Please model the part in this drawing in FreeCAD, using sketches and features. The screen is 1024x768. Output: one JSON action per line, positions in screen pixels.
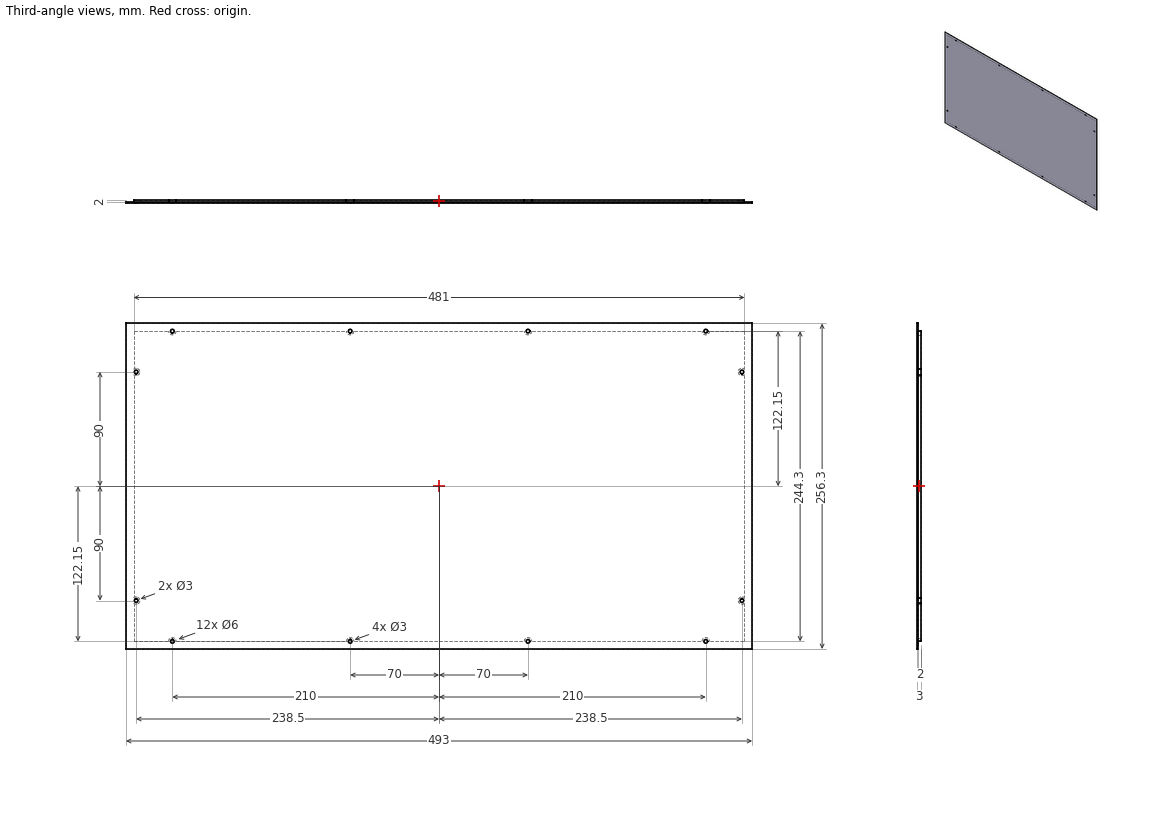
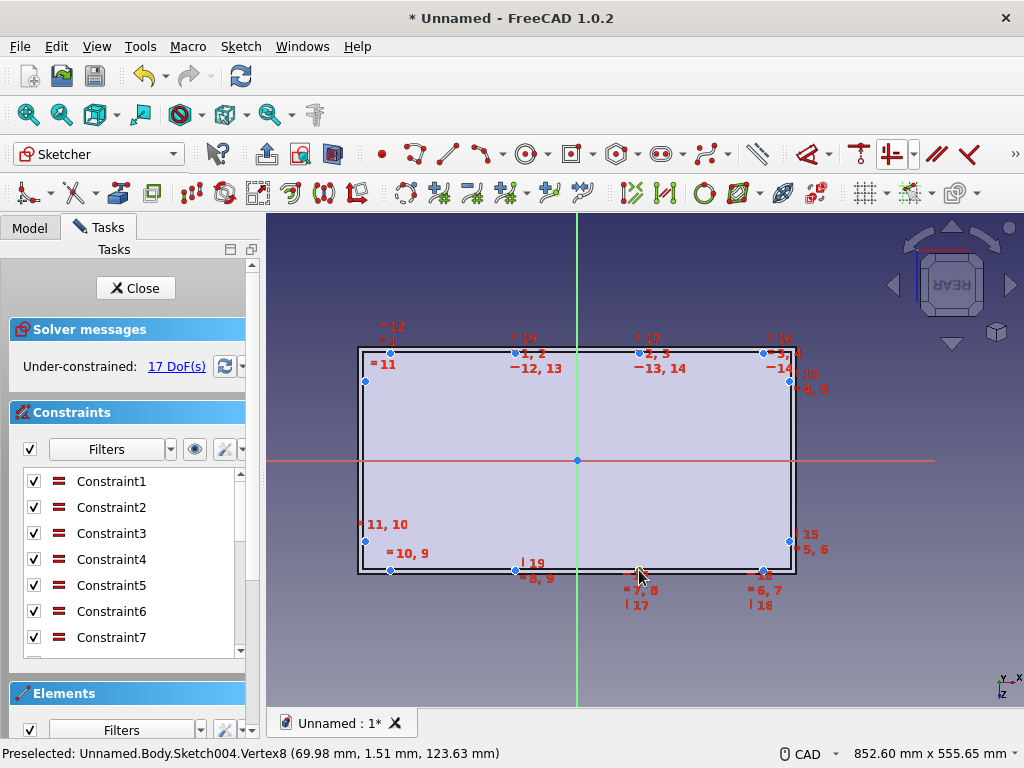
{"action": "left_click", "coordinate": [515, 570]}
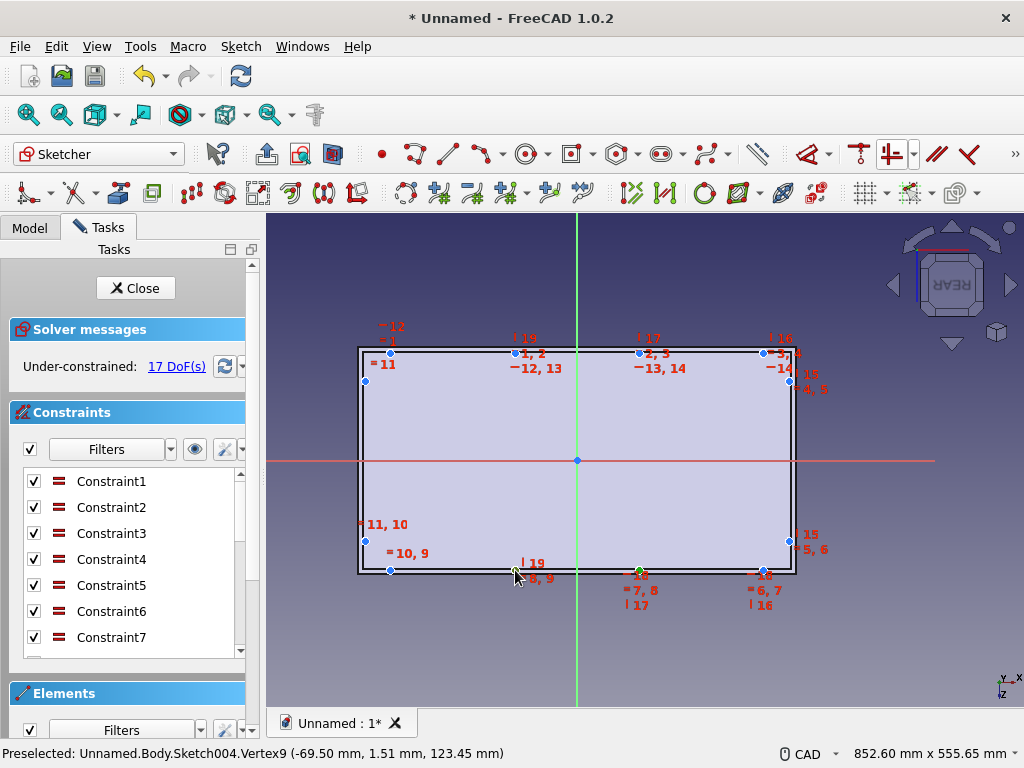
{"action": "left_click", "coordinate": [914, 154]}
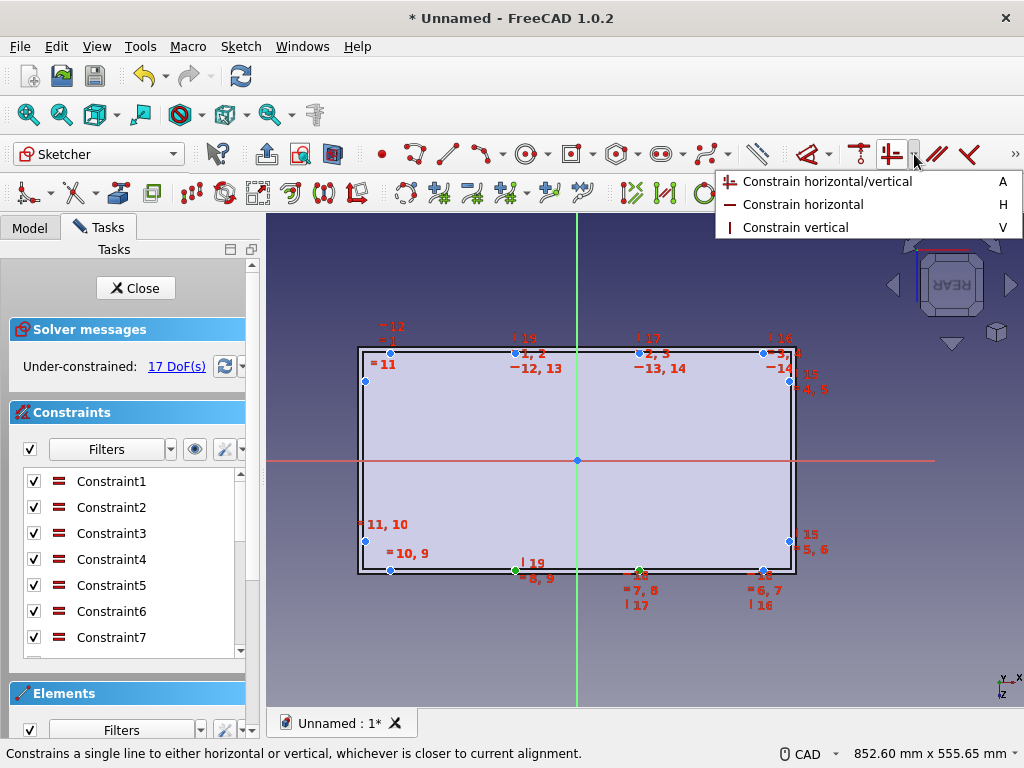
{"action": "left_click", "coordinate": [869, 204]}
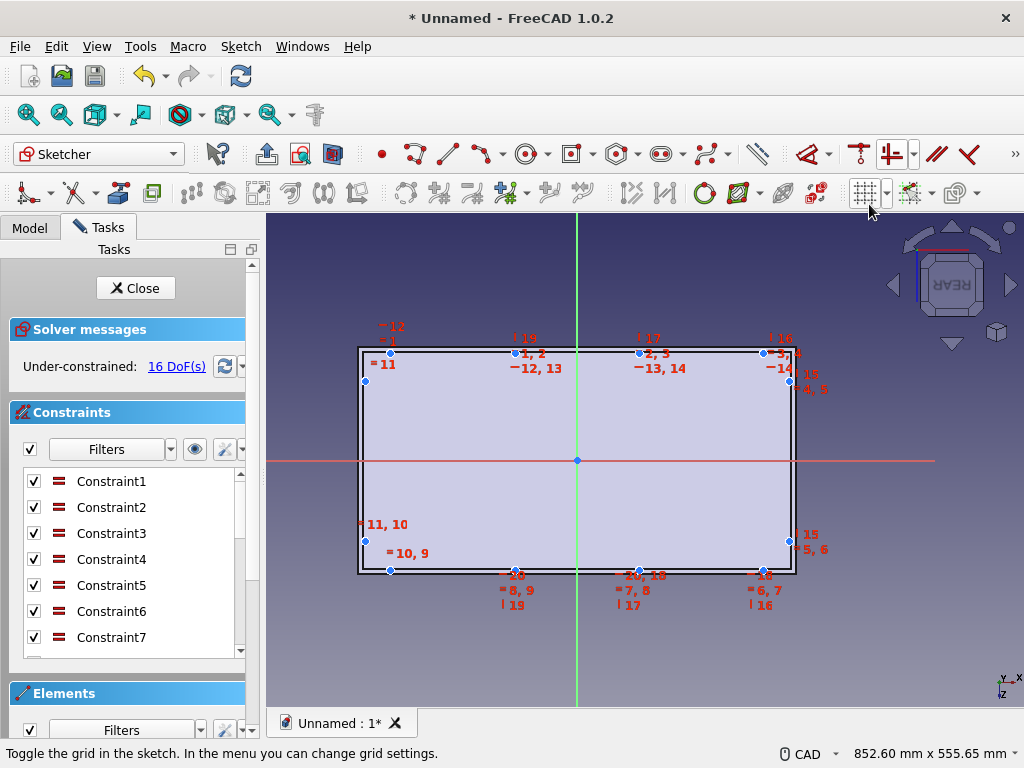
{"action": "left_click", "coordinate": [390, 353]}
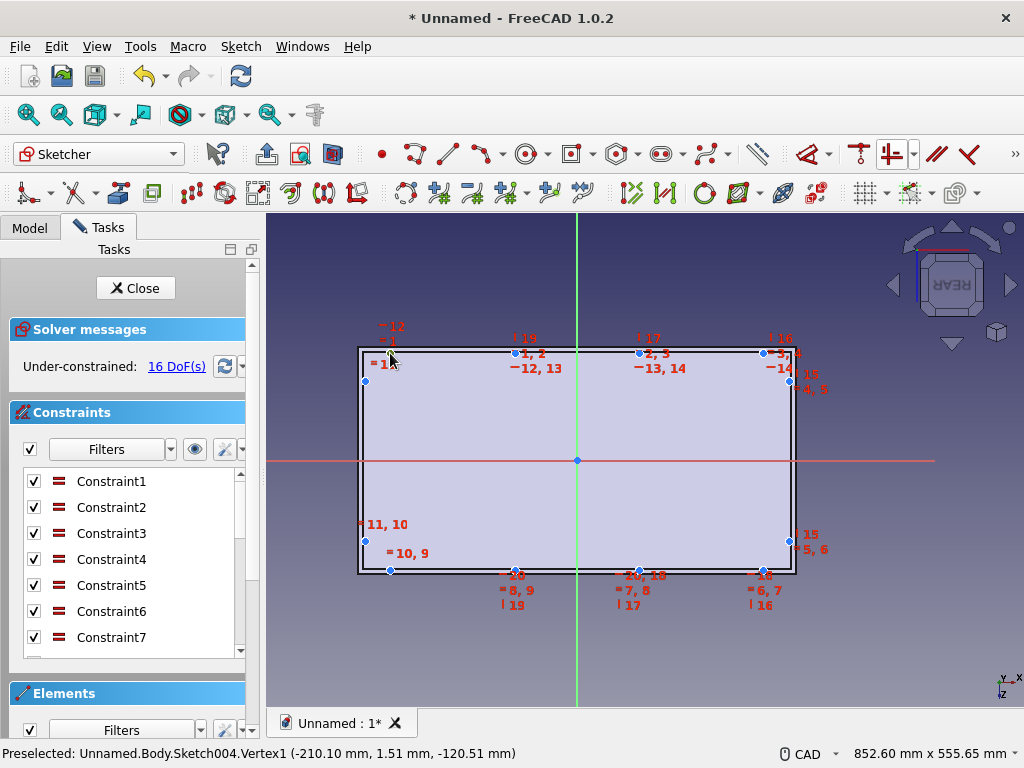
{"action": "left_click", "coordinate": [390, 570]}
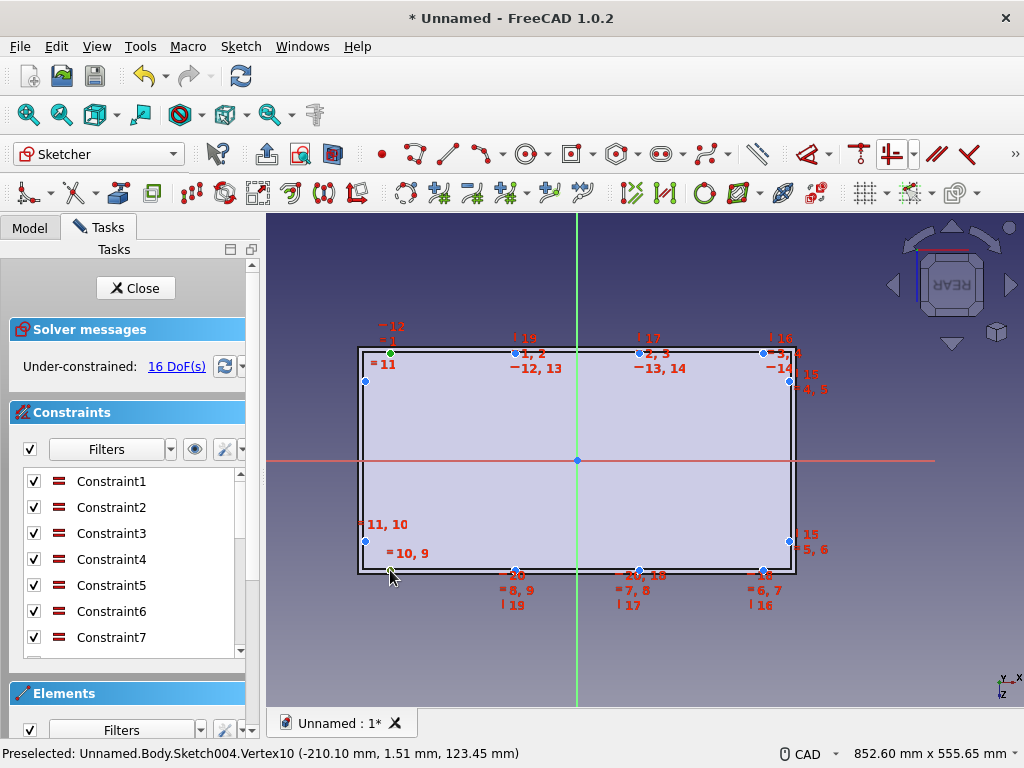
{"action": "left_click", "coordinate": [914, 154]}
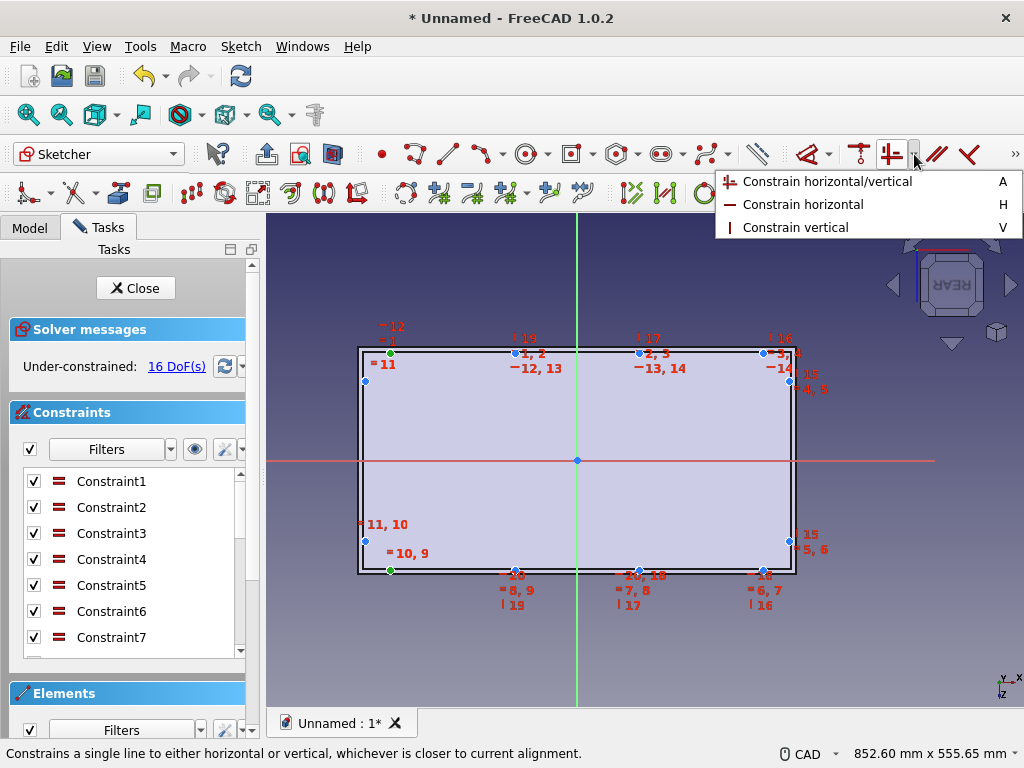
{"action": "left_click", "coordinate": [869, 228]}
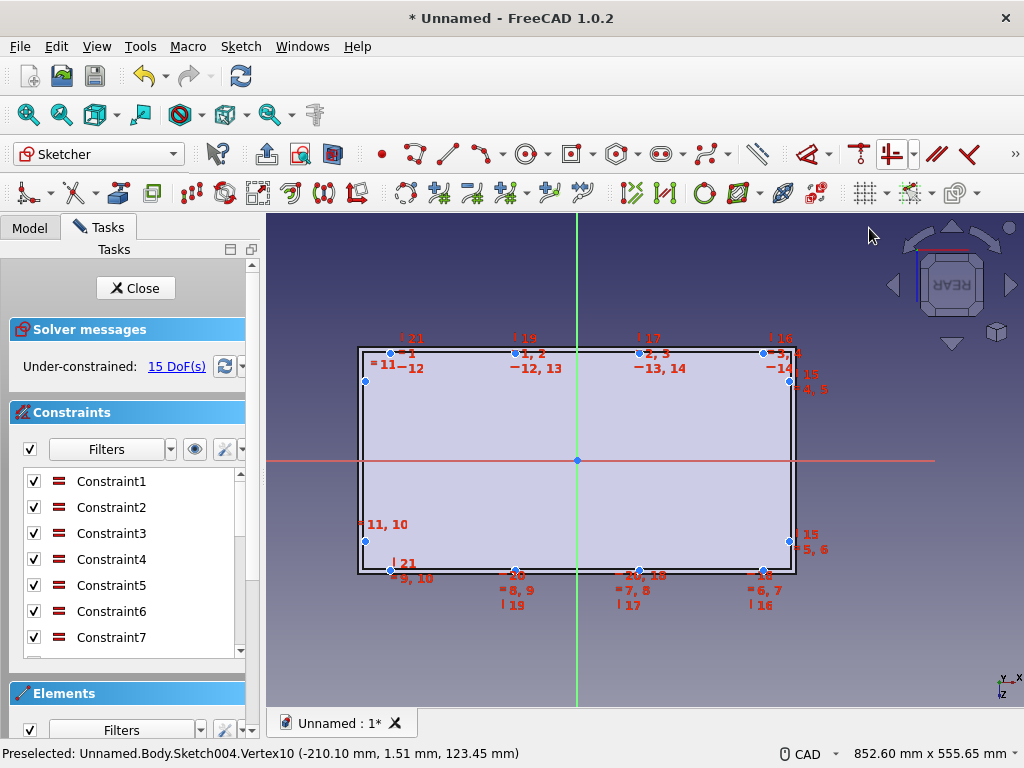
{"action": "scroll", "coordinate": [515, 570], "scroll_direction": "up", "scroll_amount": 4}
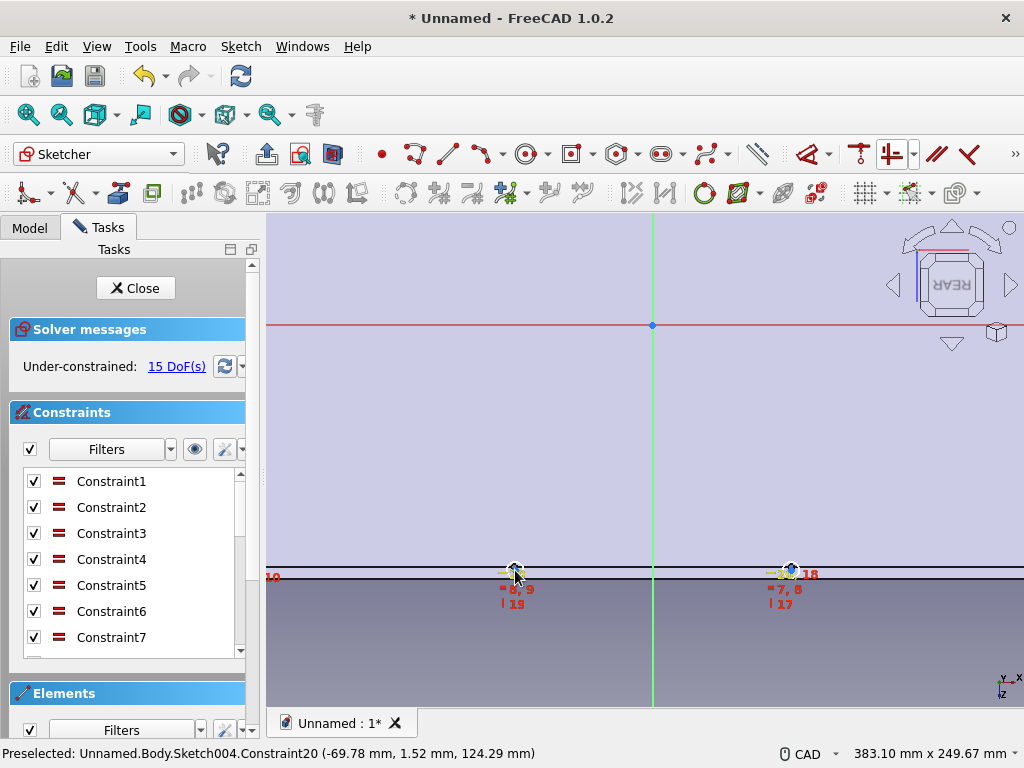
{"action": "scroll", "coordinate": [515, 570], "scroll_direction": "up", "scroll_amount": 4}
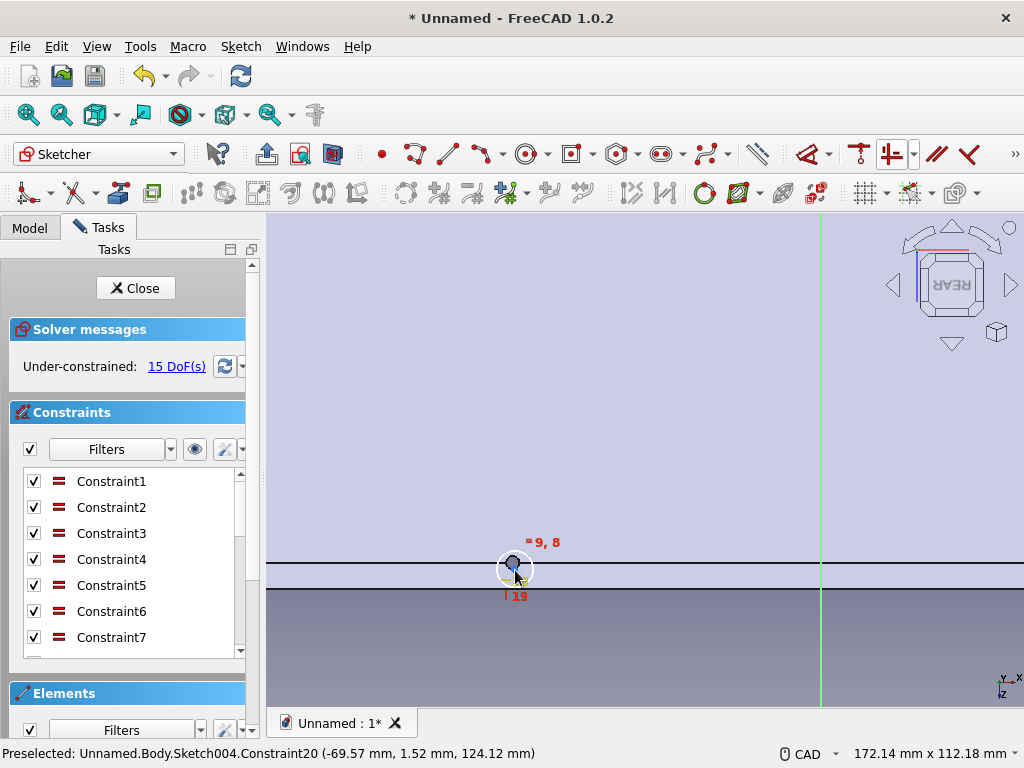
{"action": "left_click", "coordinate": [515, 569]}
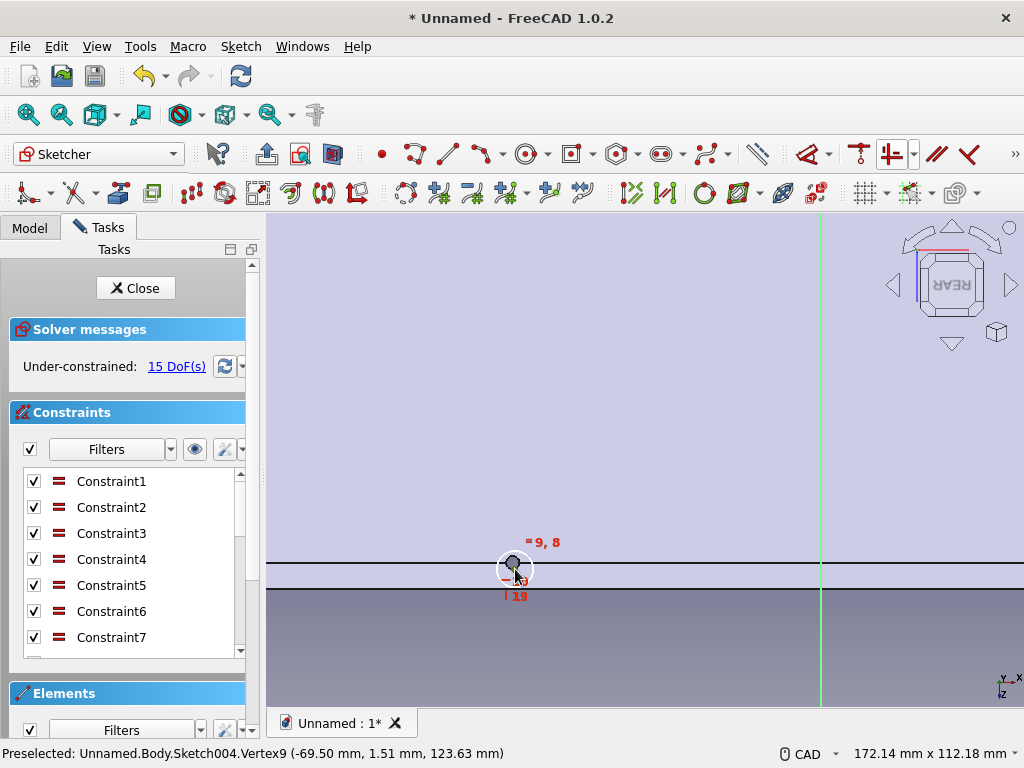
{"action": "scroll", "coordinate": [515, 570], "scroll_direction": "down", "scroll_amount": 8}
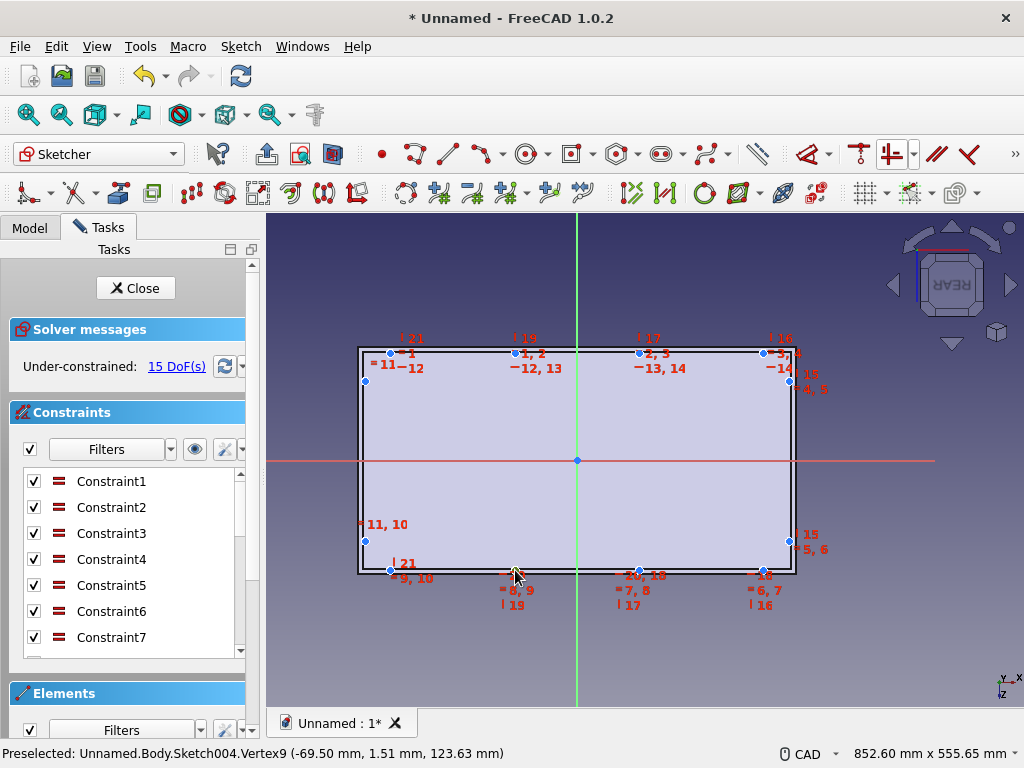
{"action": "scroll", "coordinate": [390, 570], "scroll_direction": "up", "scroll_amount": 4}